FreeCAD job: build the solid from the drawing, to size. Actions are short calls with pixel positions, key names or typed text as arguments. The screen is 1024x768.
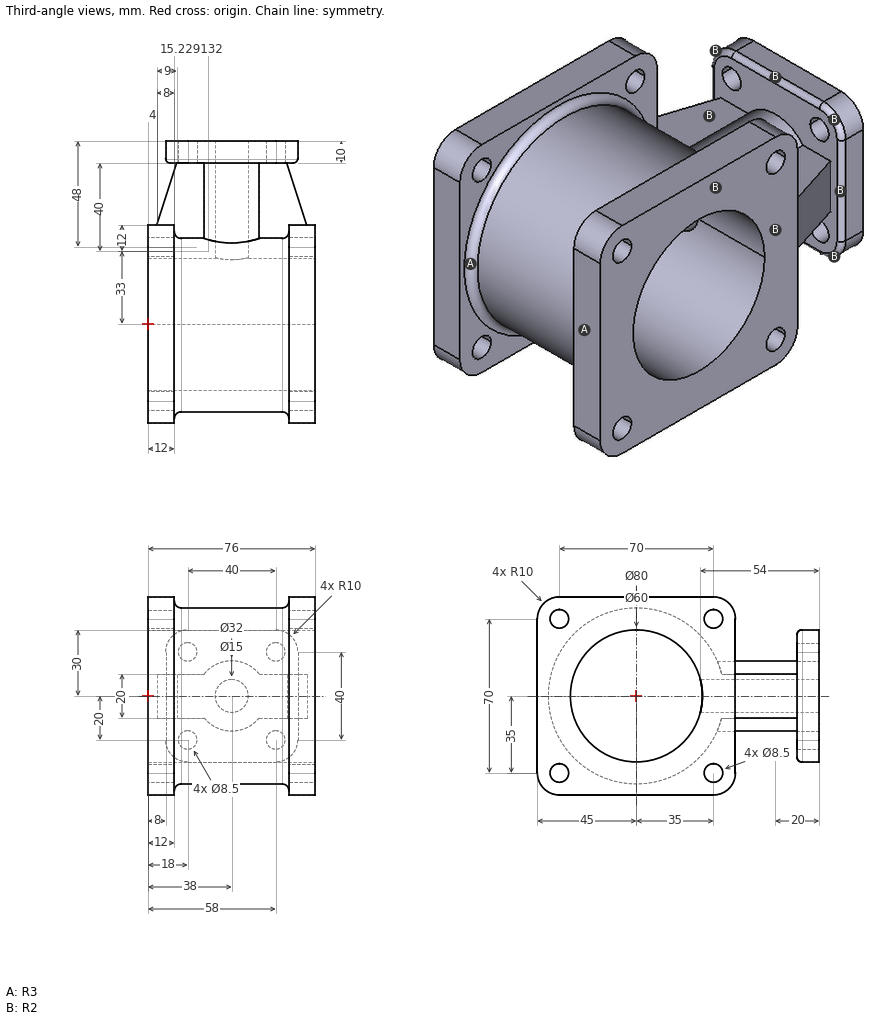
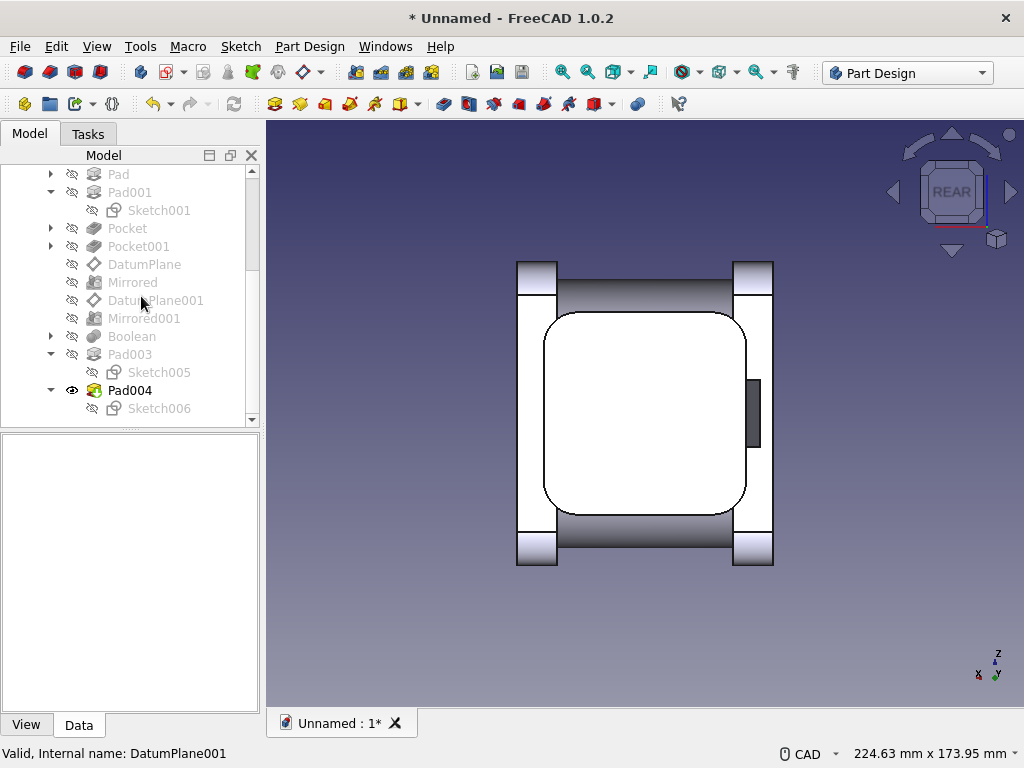
scroll(141, 296, up, 15)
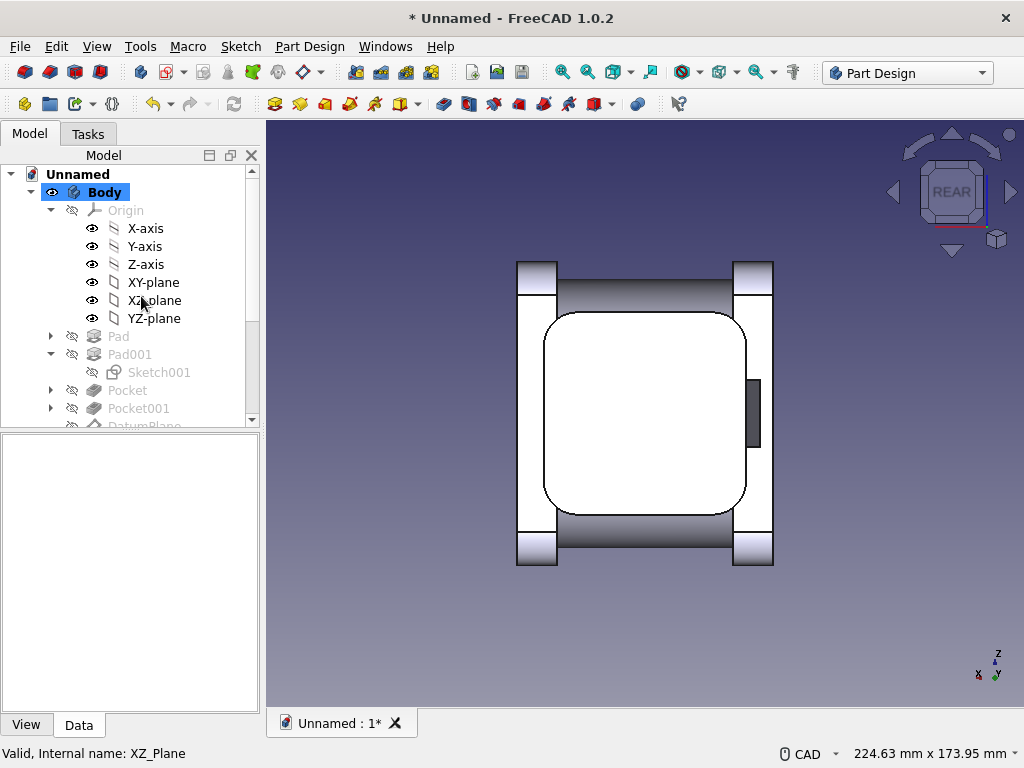
click(137, 318)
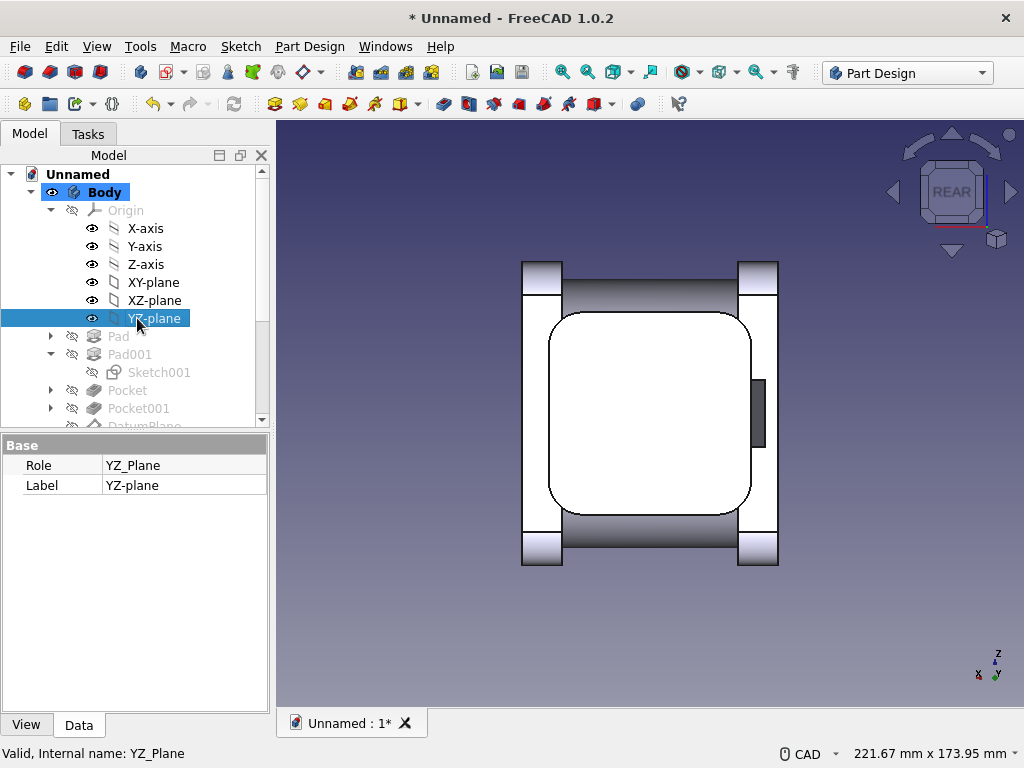
click(302, 72)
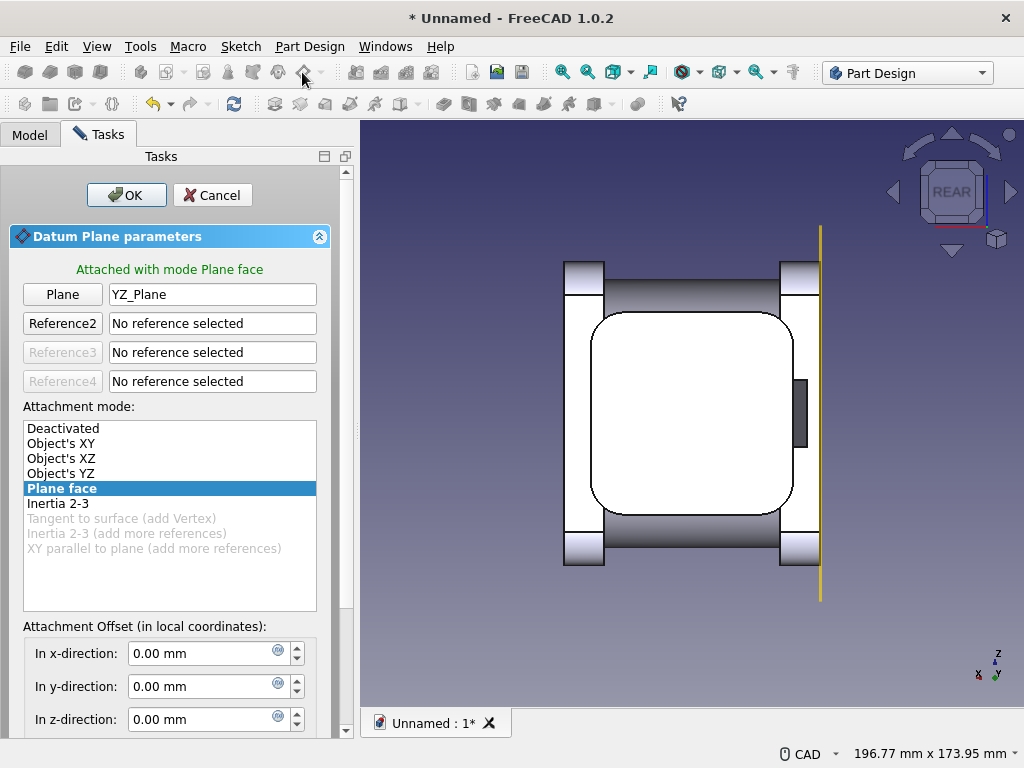
triple_click(210, 720)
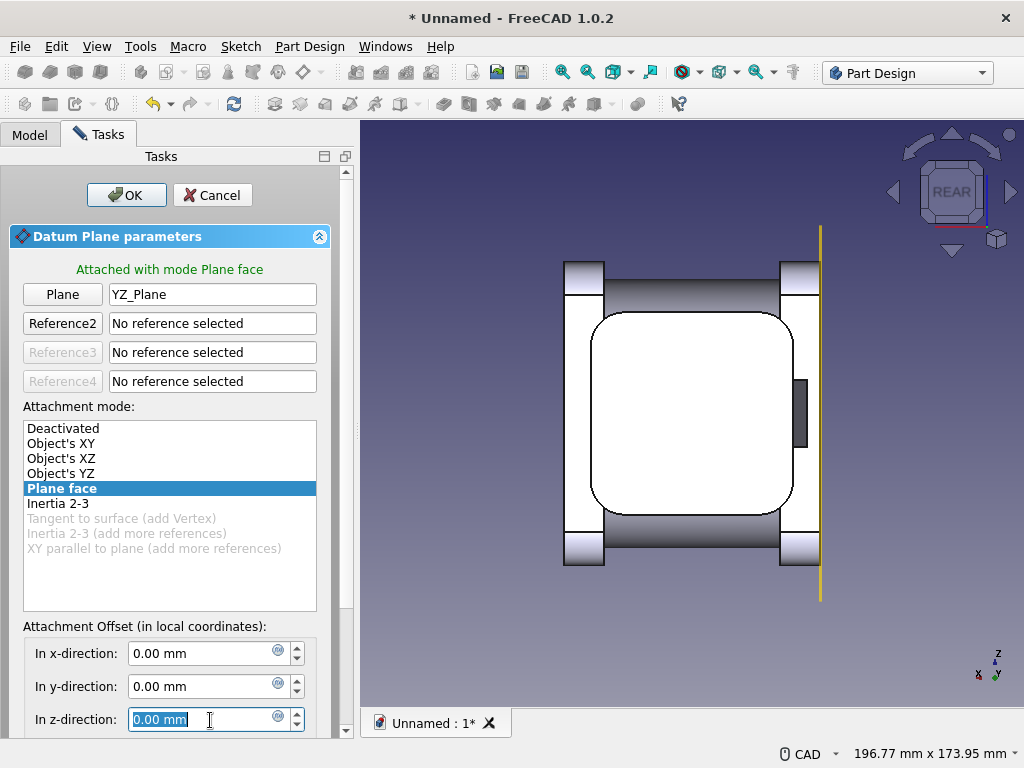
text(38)
key(Tab)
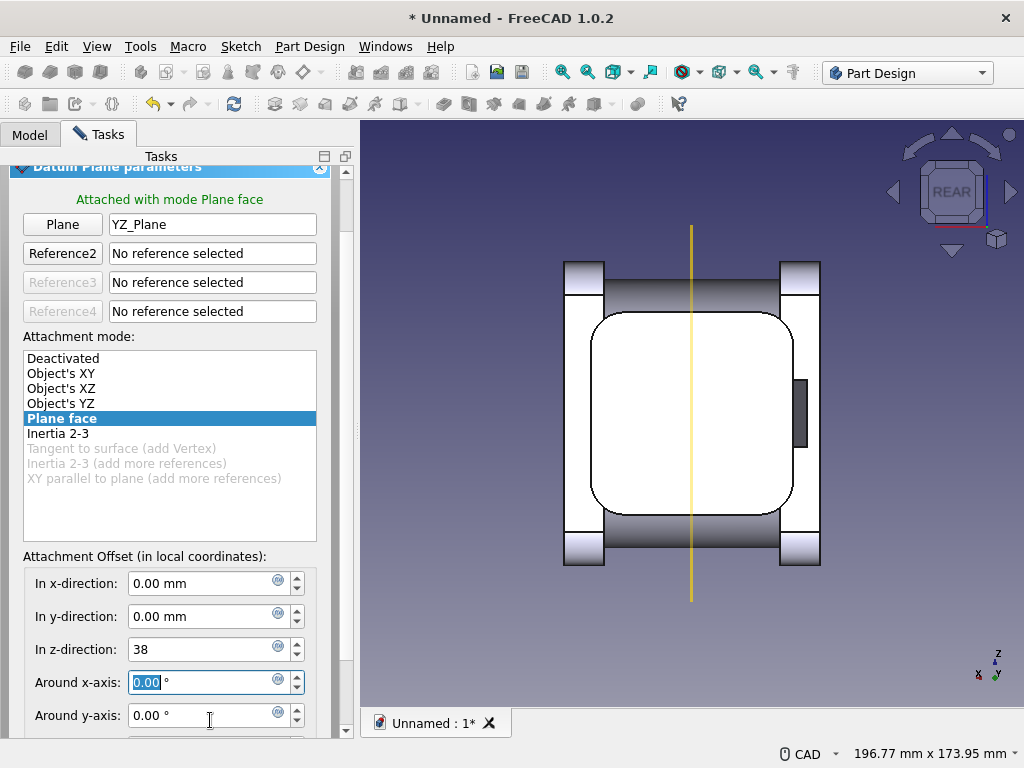
scroll(346, 452, up, 2)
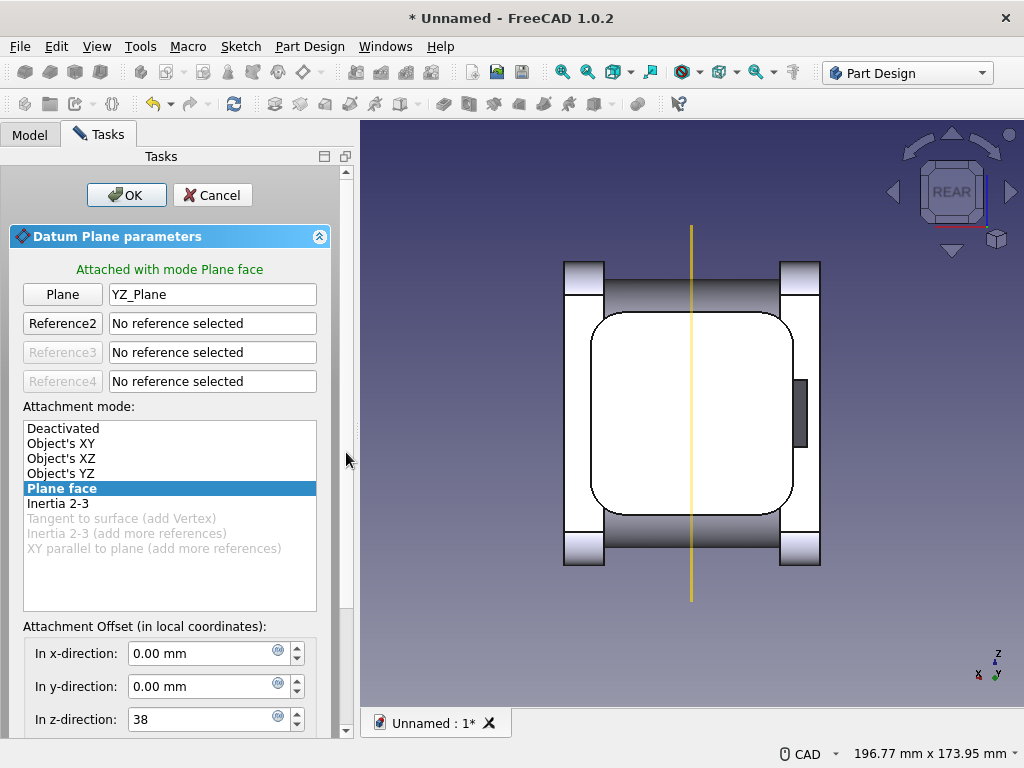
click(127, 195)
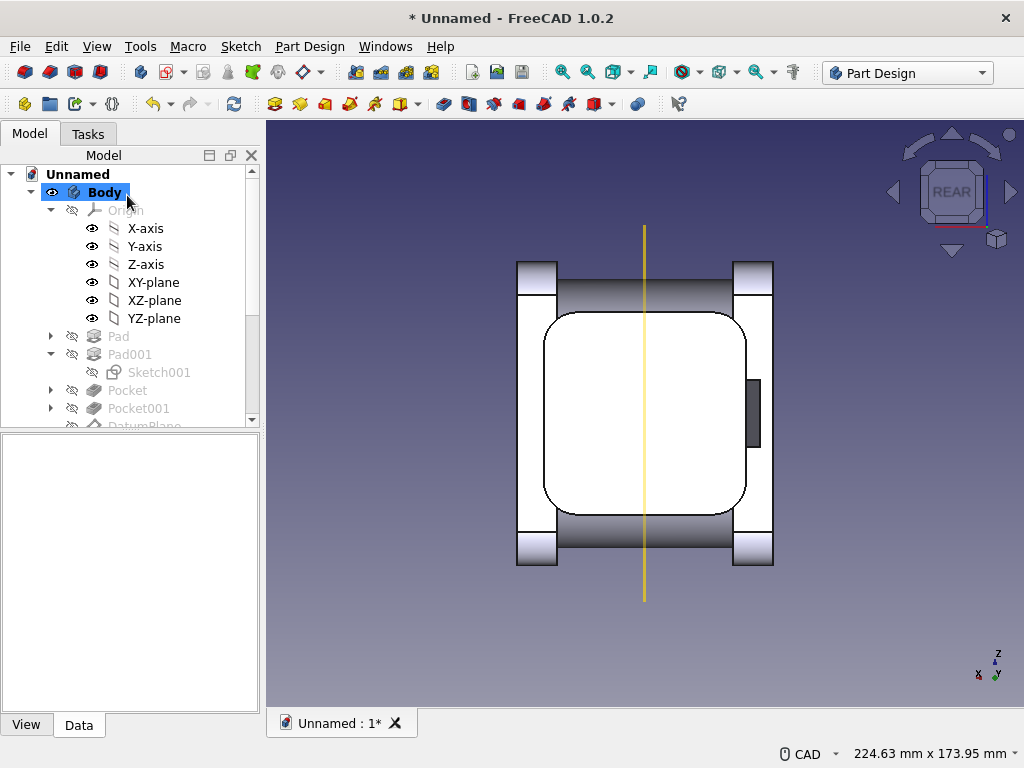
scroll(101, 296, down, 3)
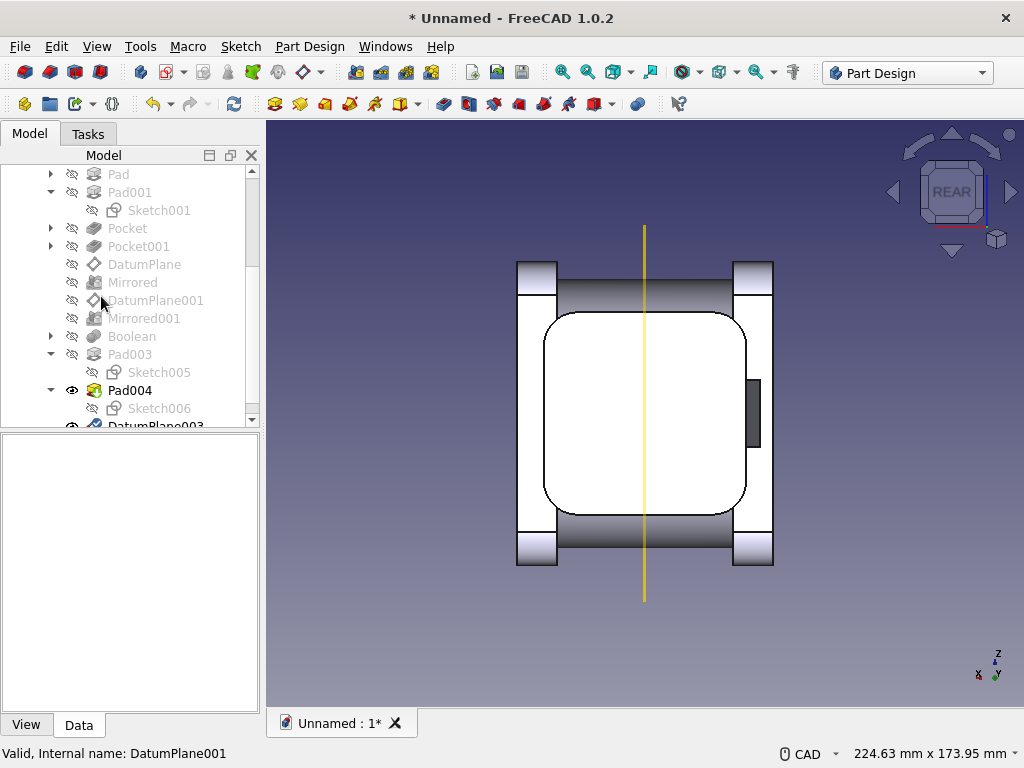
click(117, 390)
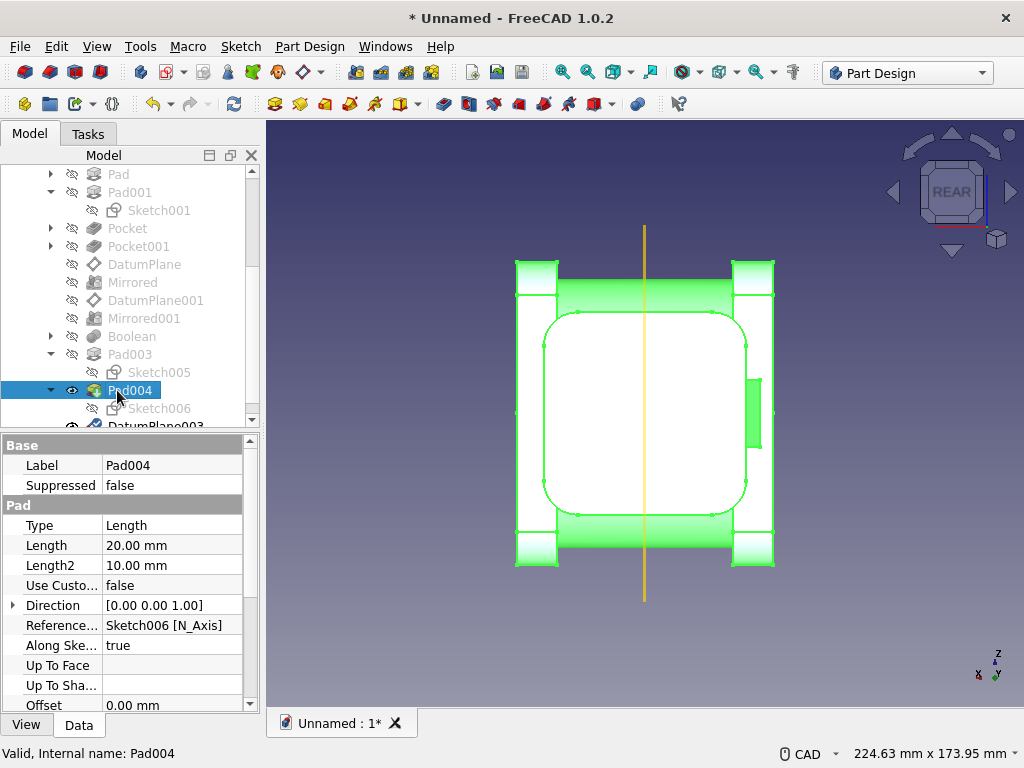
click(356, 72)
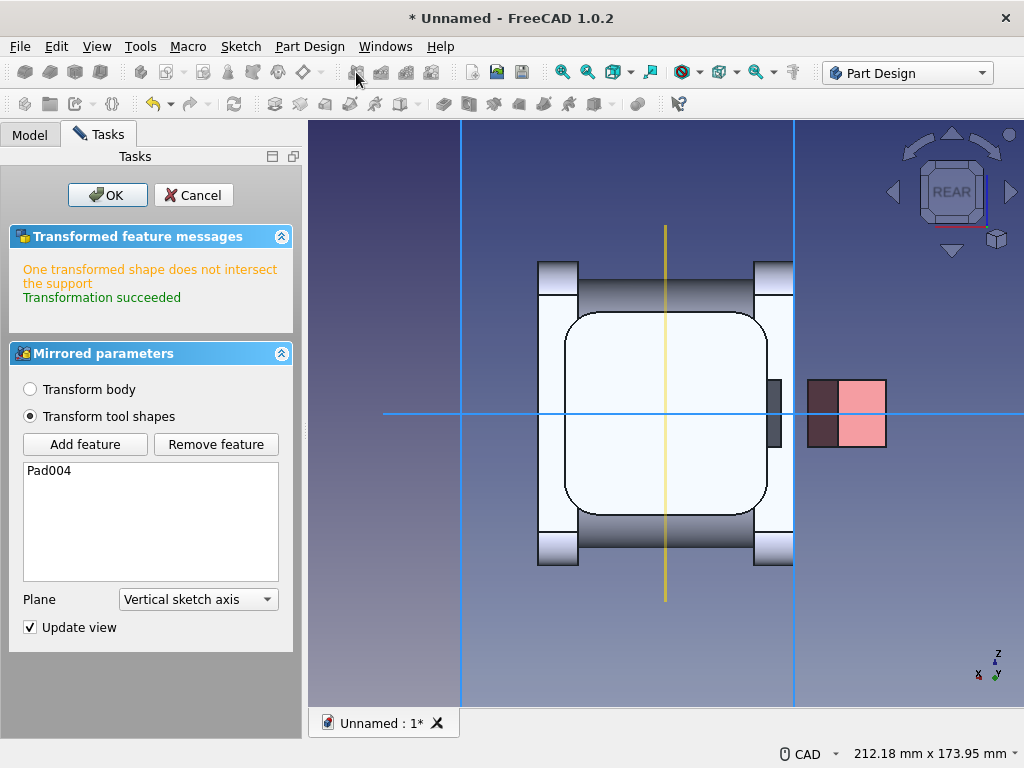
click(199, 600)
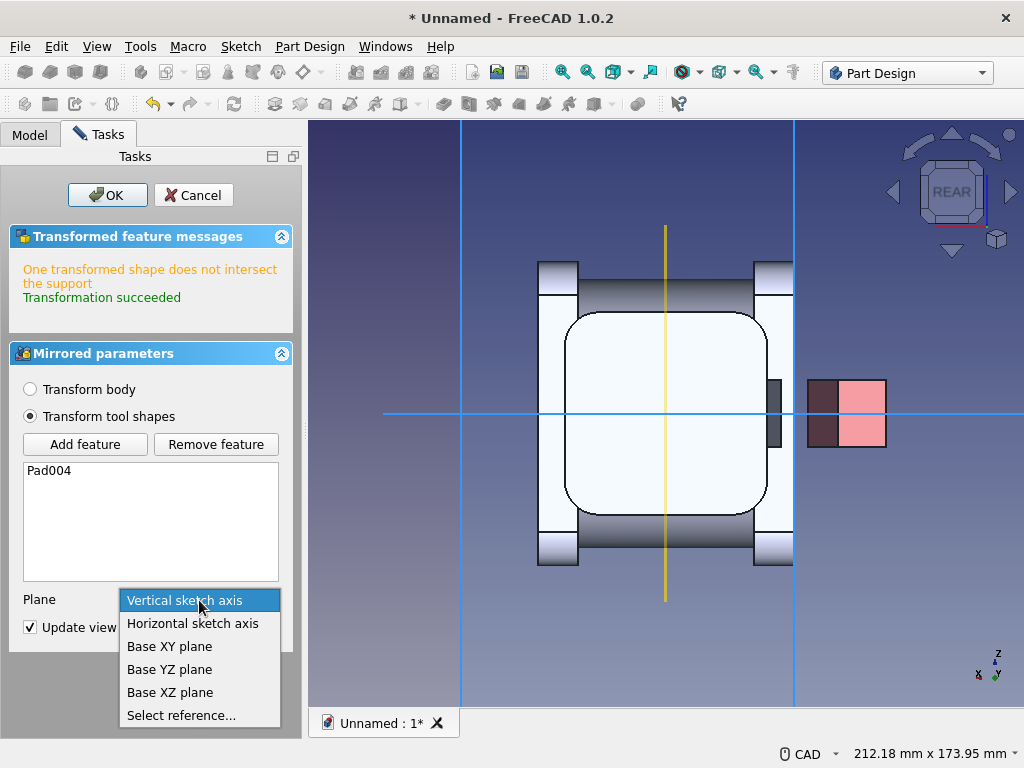
click(198, 716)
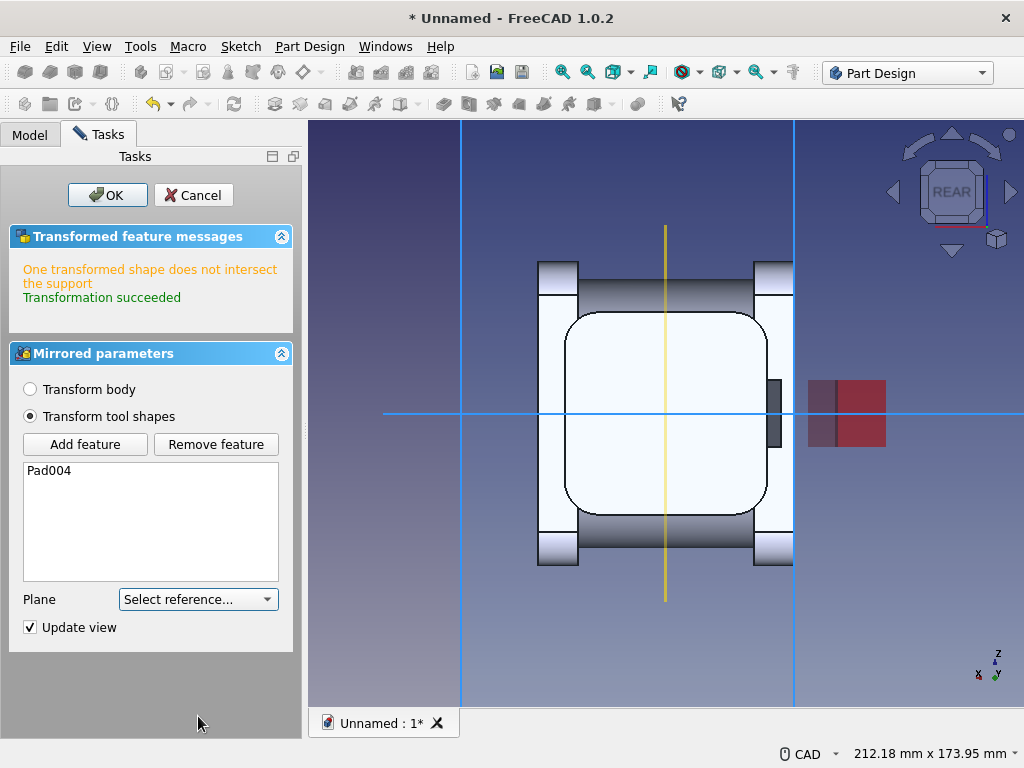
click(30, 134)